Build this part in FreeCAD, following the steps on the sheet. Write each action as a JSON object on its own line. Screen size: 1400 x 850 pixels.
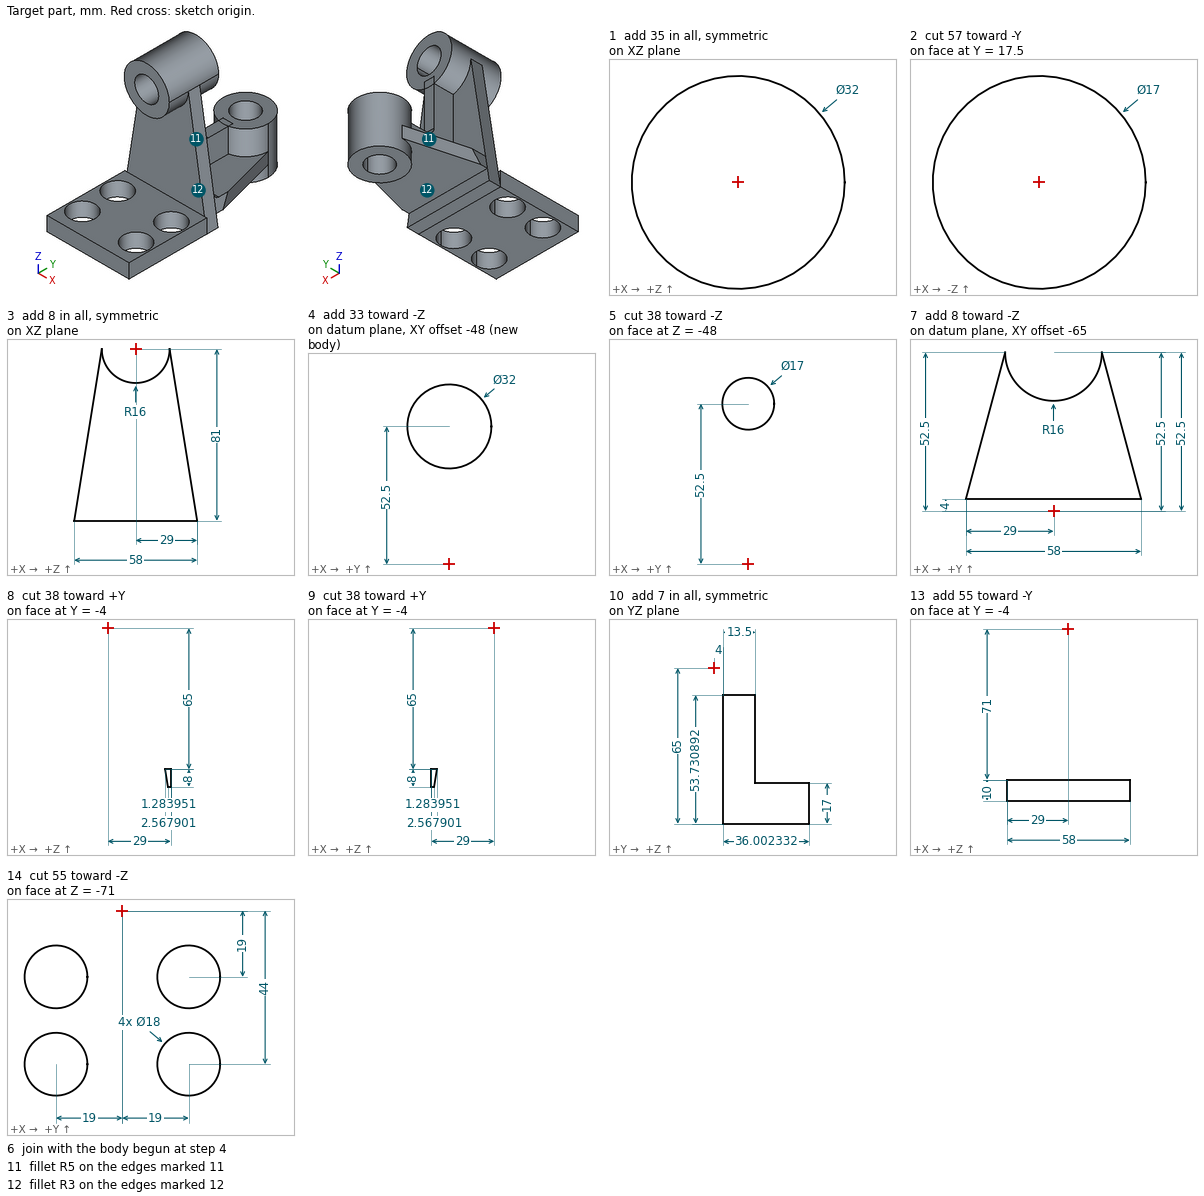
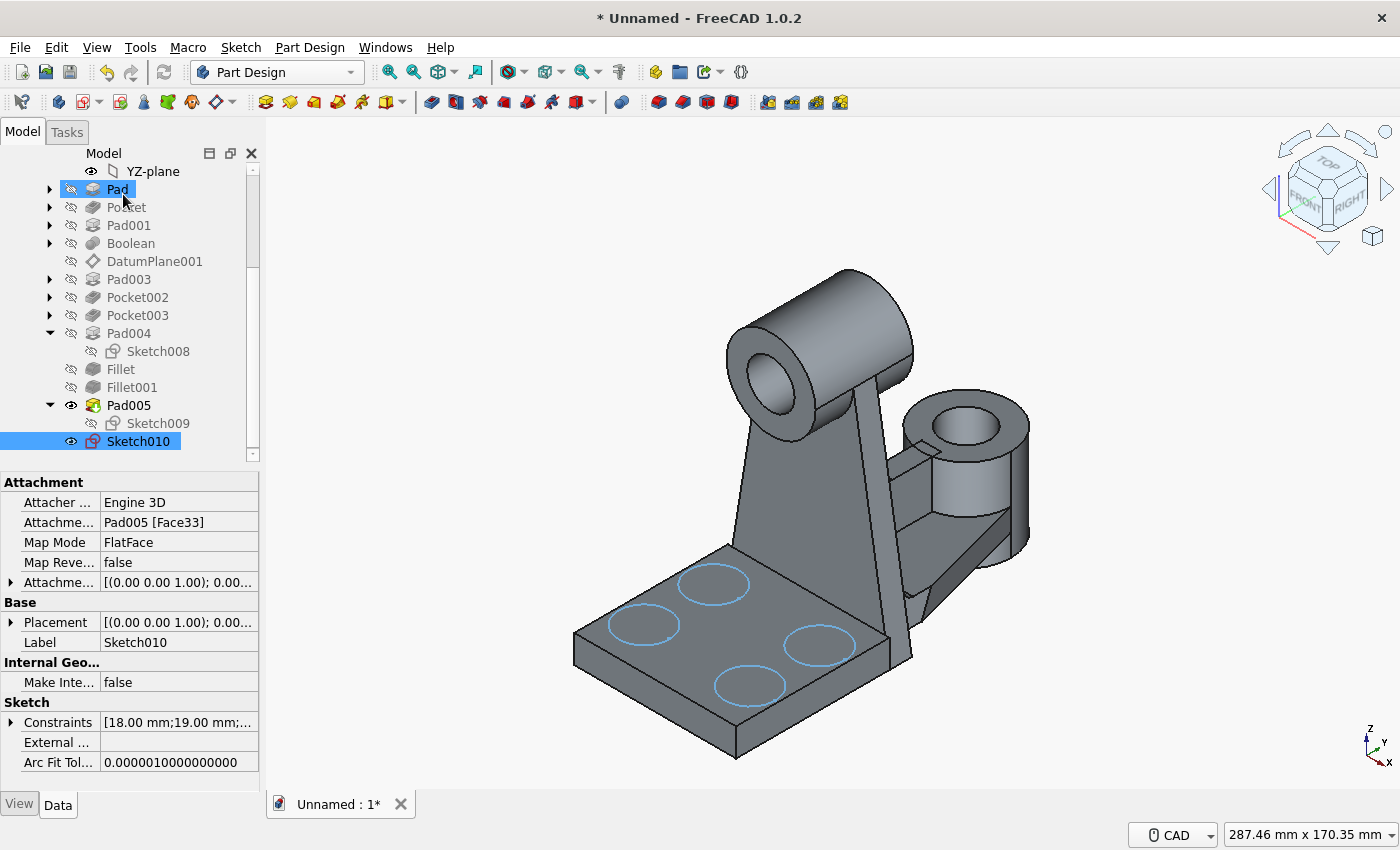
{"action": "left_click", "coordinate": [432, 102]}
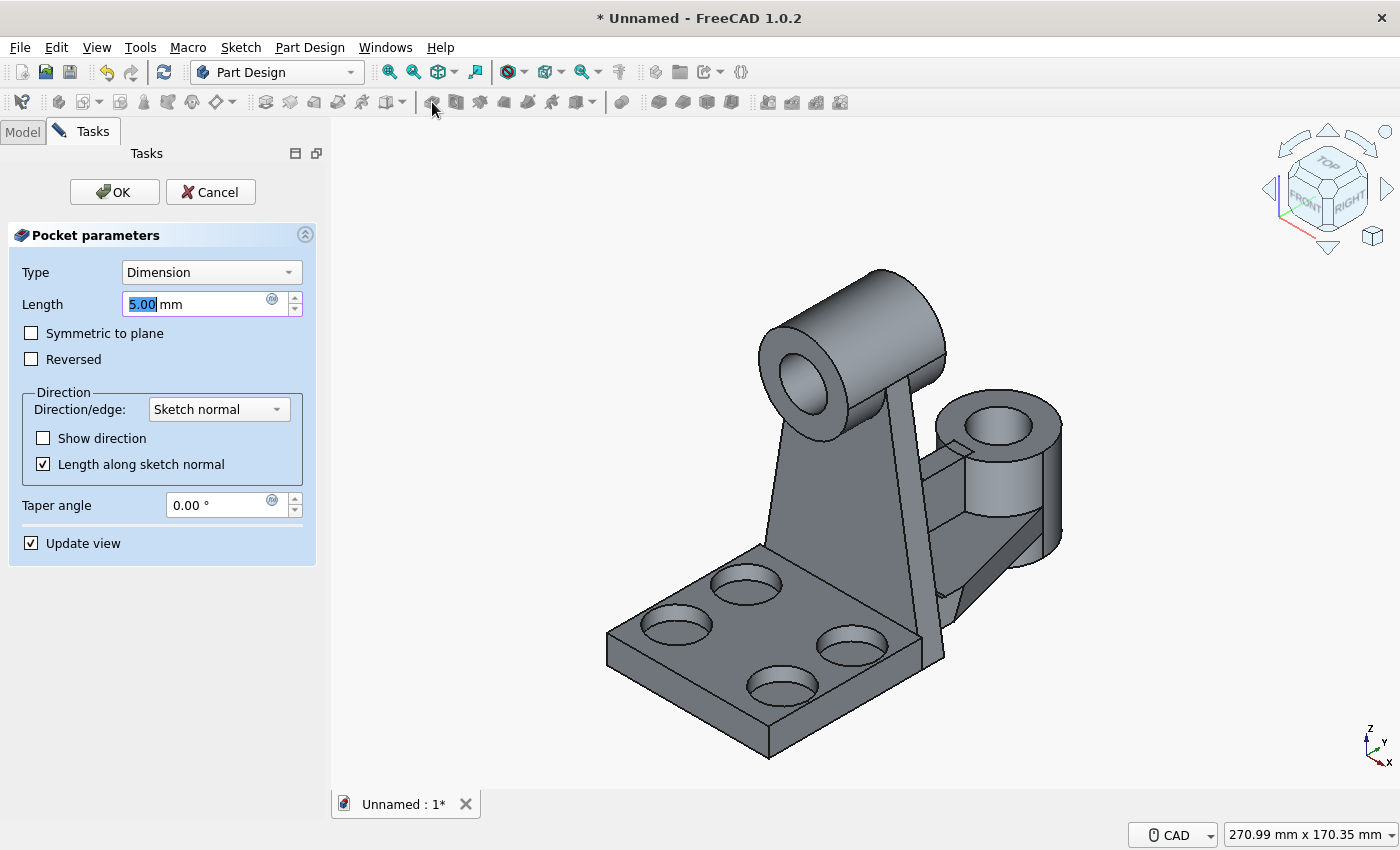
{"action": "type", "text": "55"}
{"action": "key", "text": "Tab"}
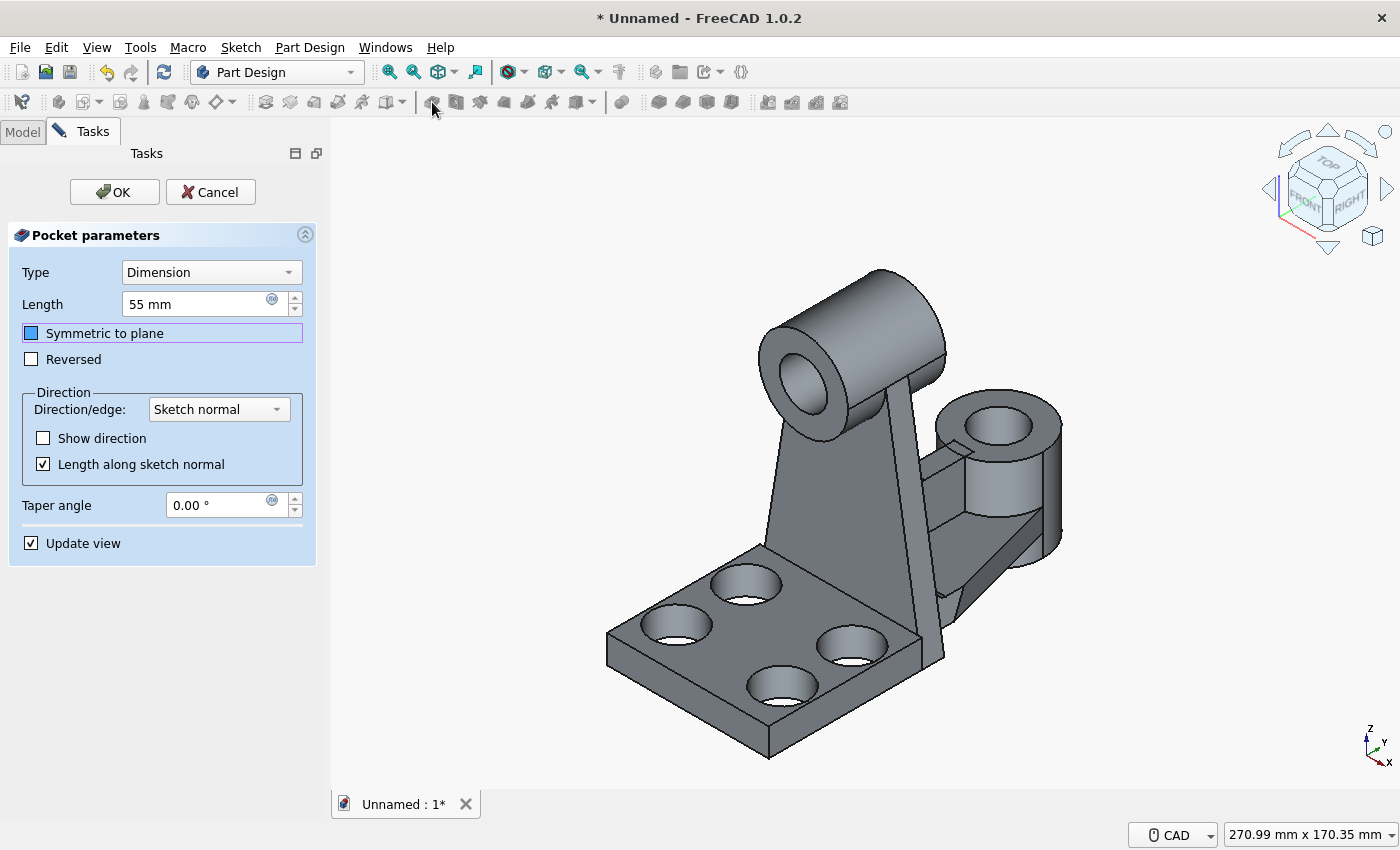
{"action": "left_click", "coordinate": [115, 192]}